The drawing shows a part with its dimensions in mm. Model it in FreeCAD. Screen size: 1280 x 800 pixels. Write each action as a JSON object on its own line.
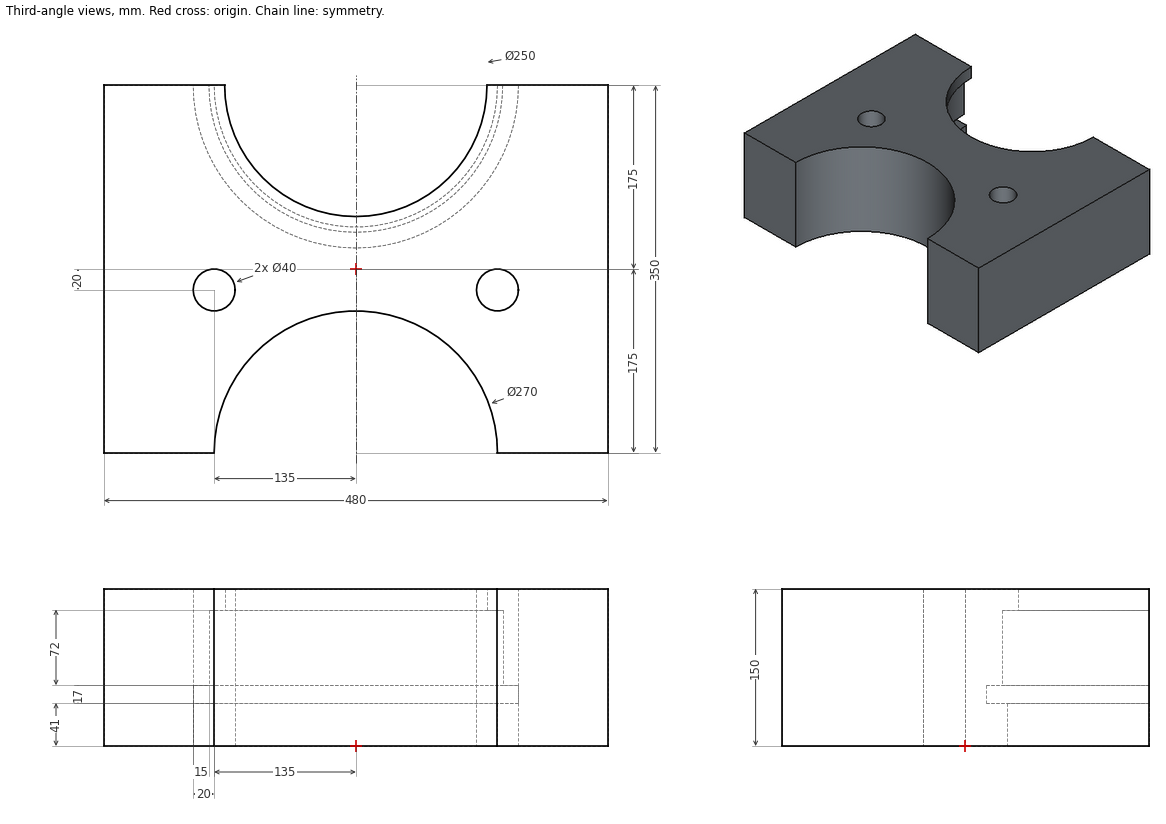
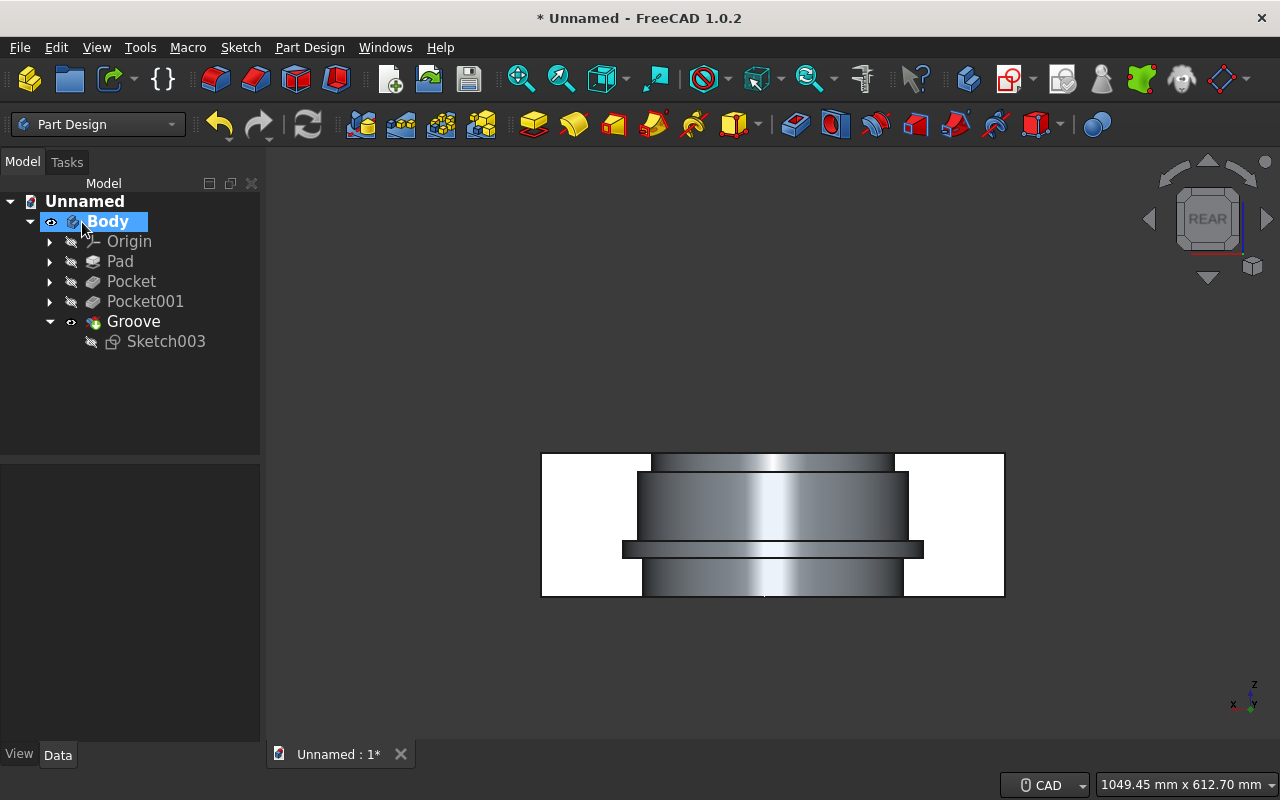
{"action": "key", "text": "0"}